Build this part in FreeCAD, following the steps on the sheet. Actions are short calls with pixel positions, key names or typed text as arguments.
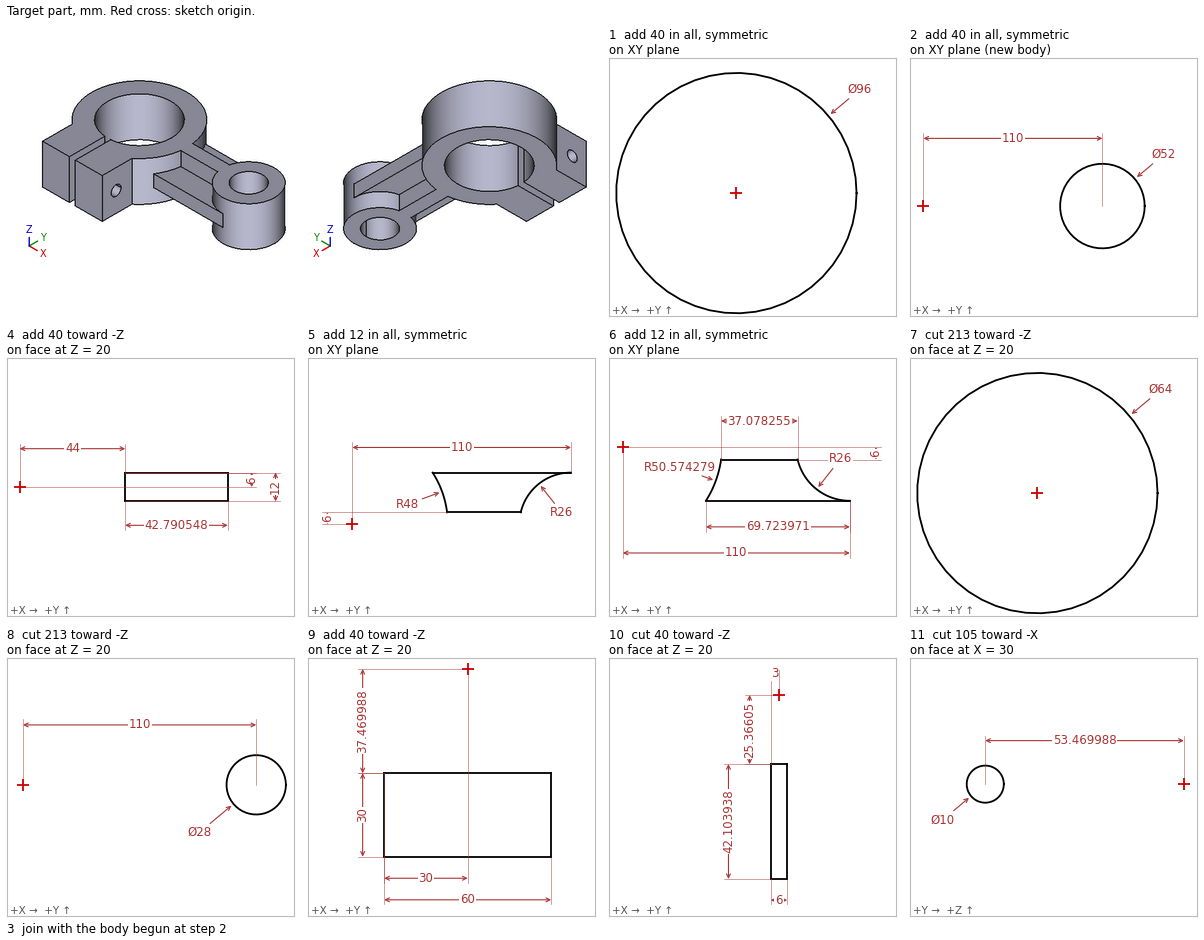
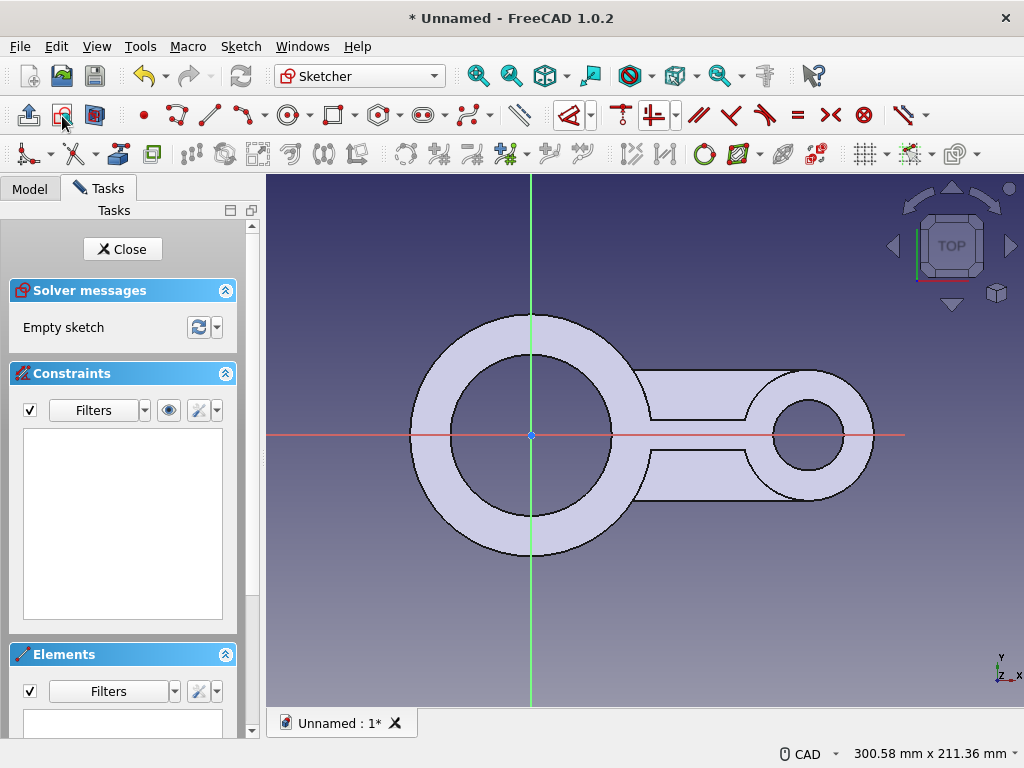
scroll(476, 618, up, 3)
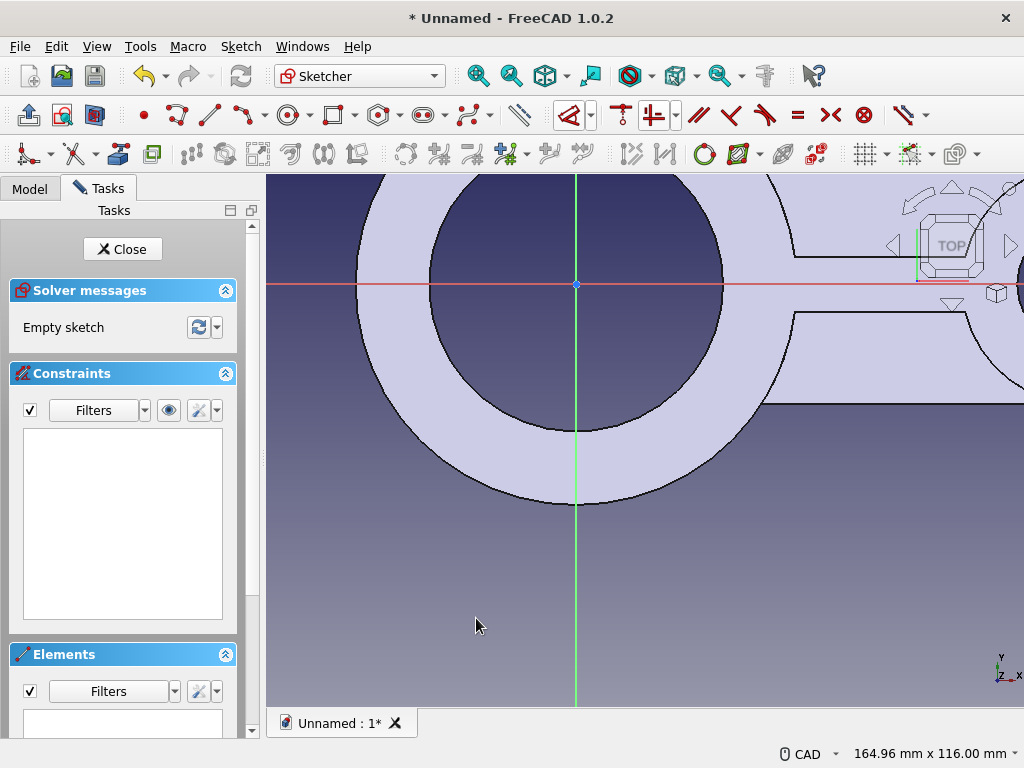
click(332, 116)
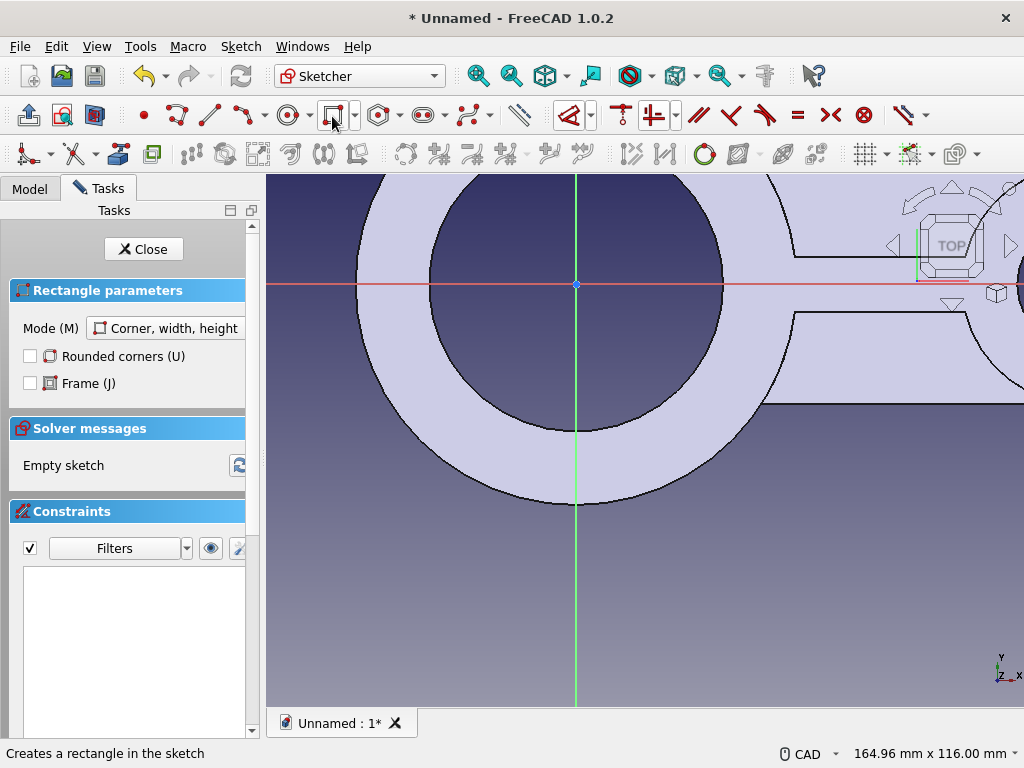
click(438, 457)
click(714, 594)
key(Escape)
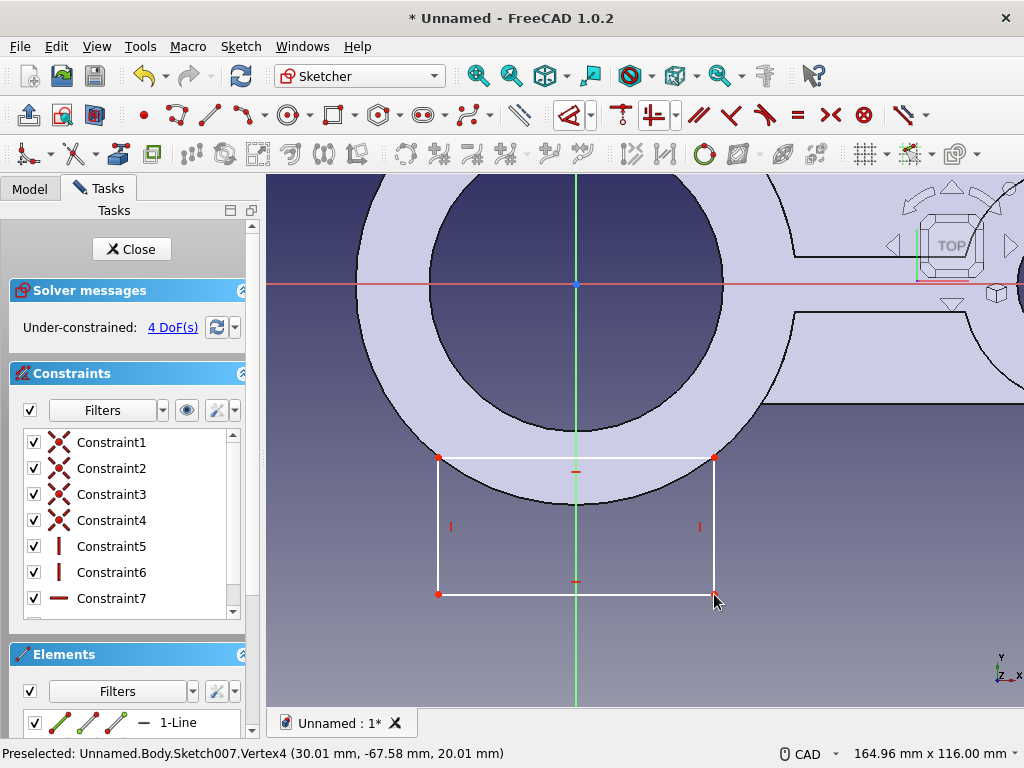
click(438, 499)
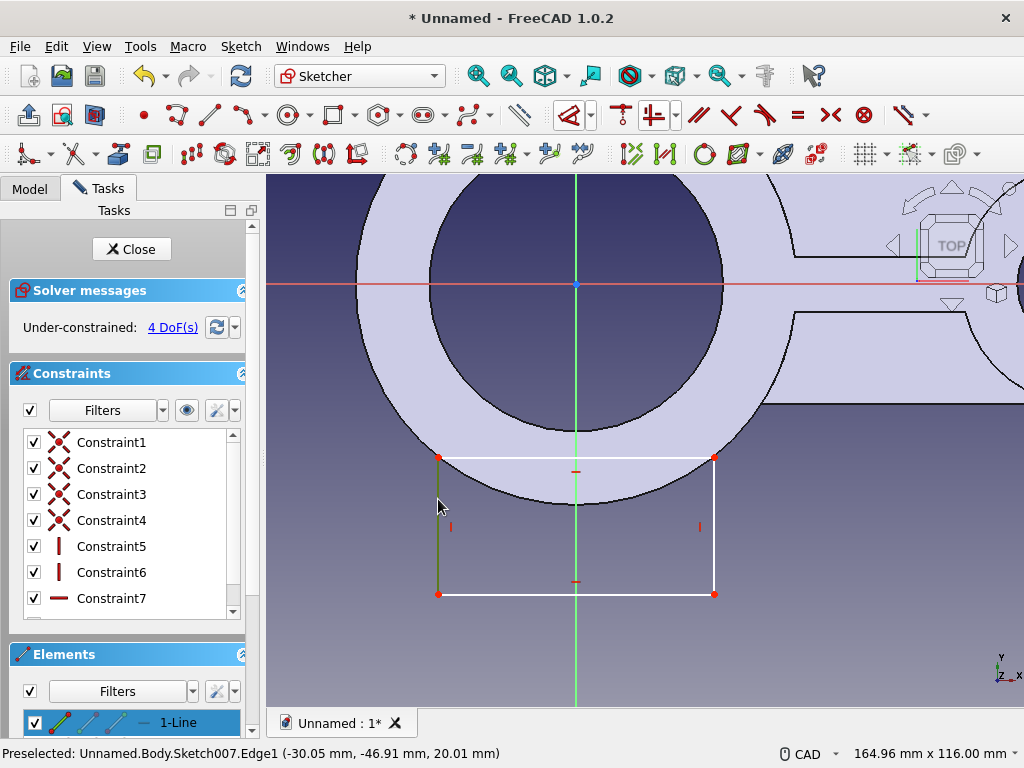
key(i)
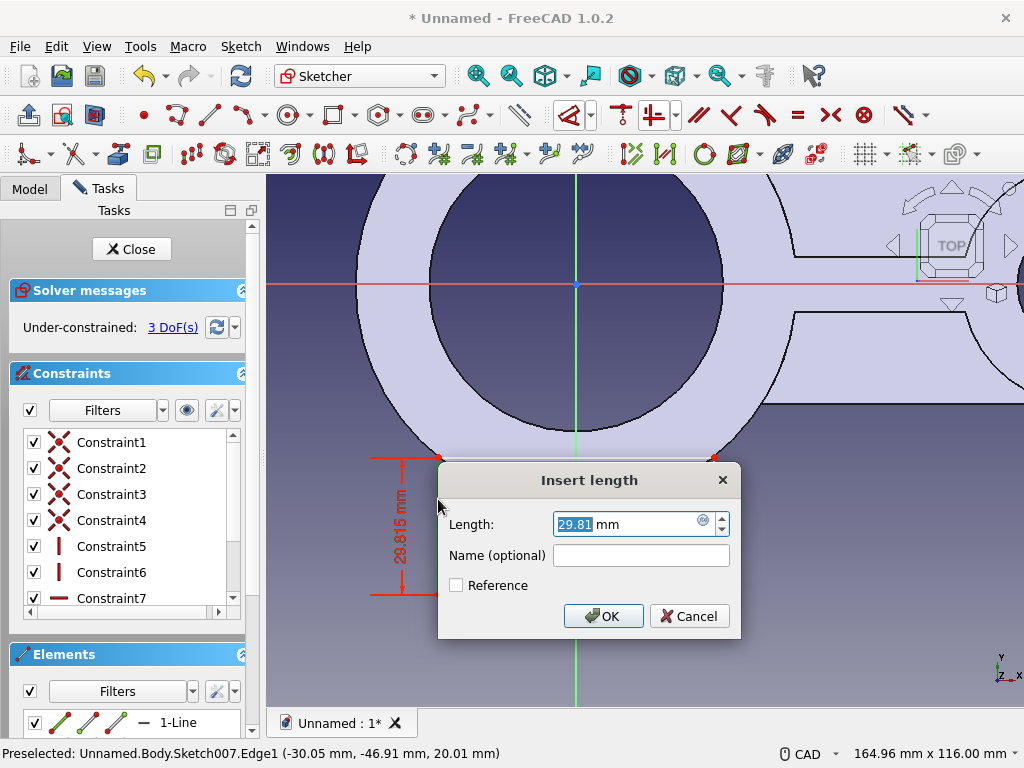
text(30)
key(Return)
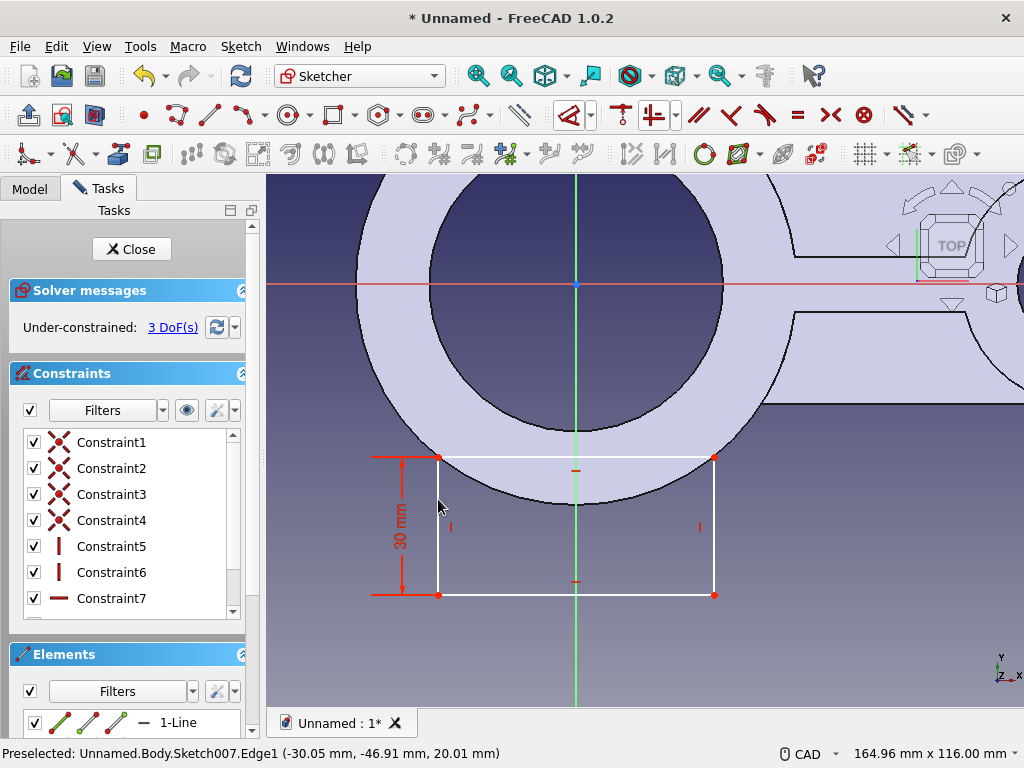
click(521, 595)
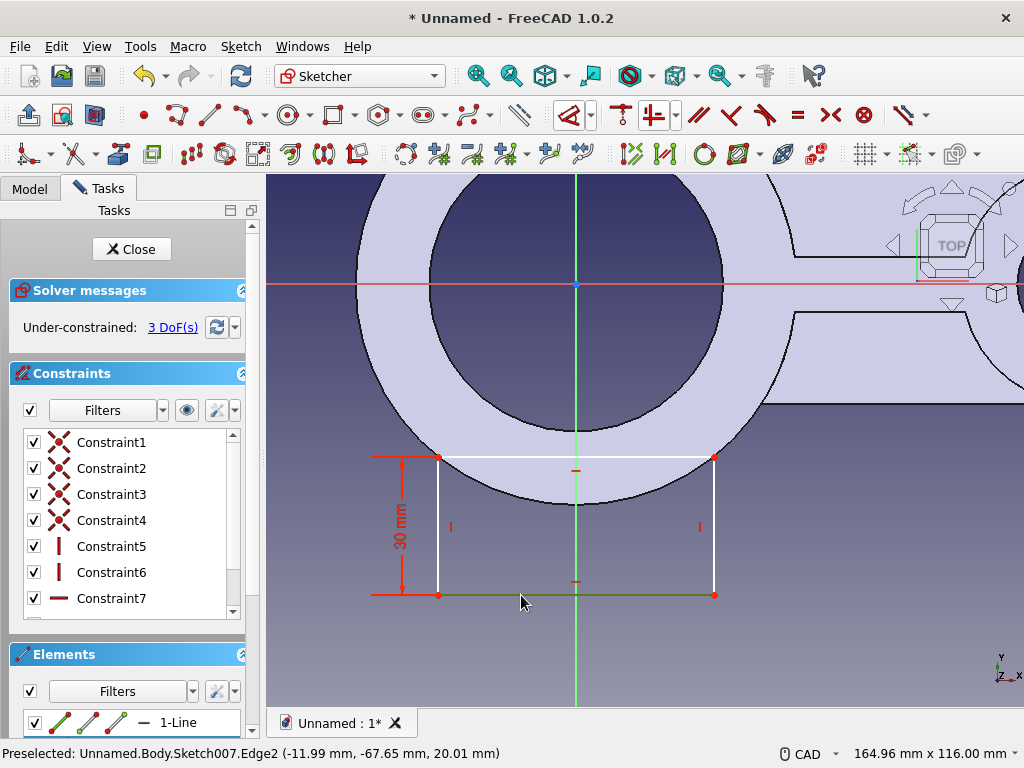
click(590, 116)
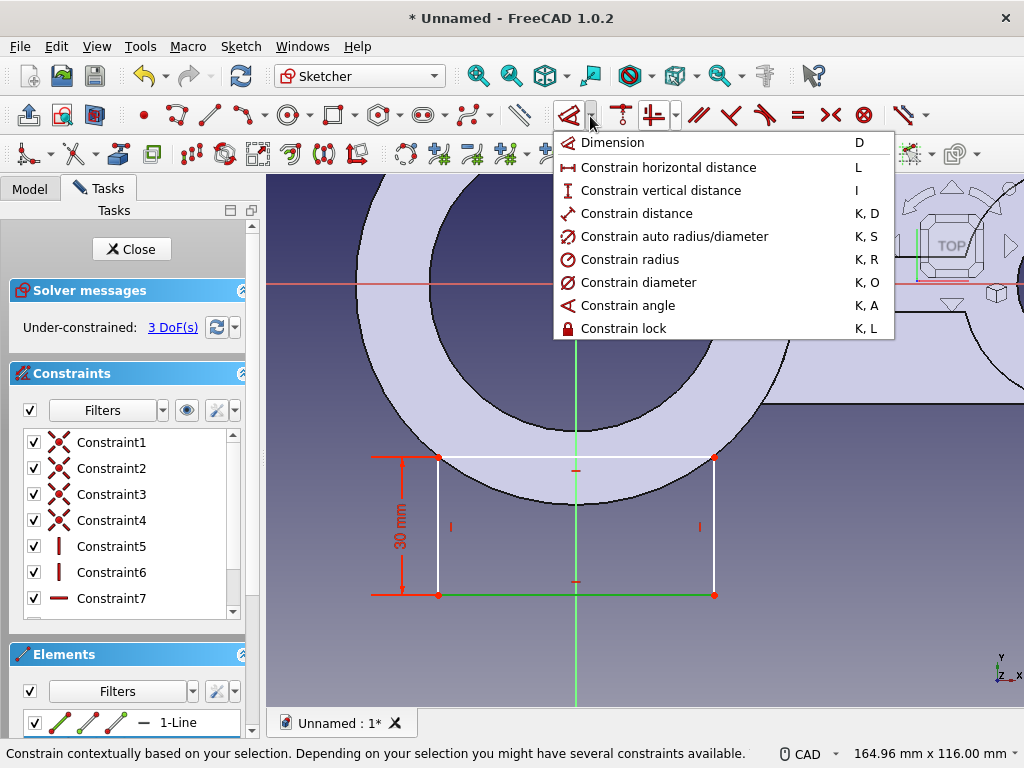
click(724, 168)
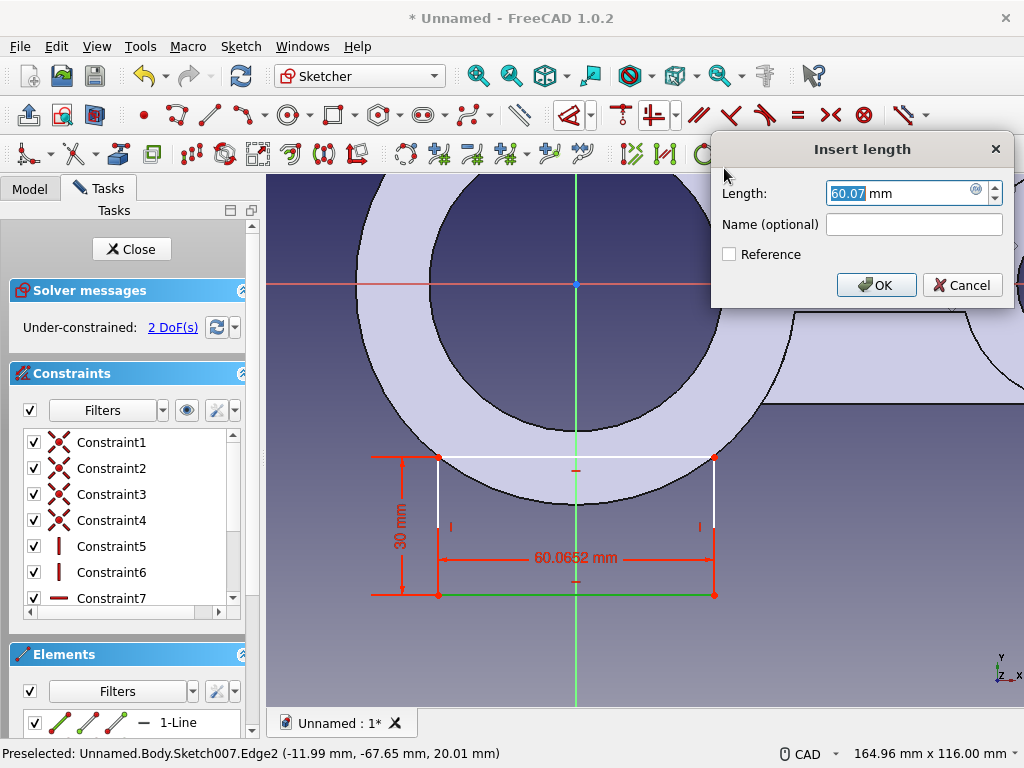
text(60)
key(Return)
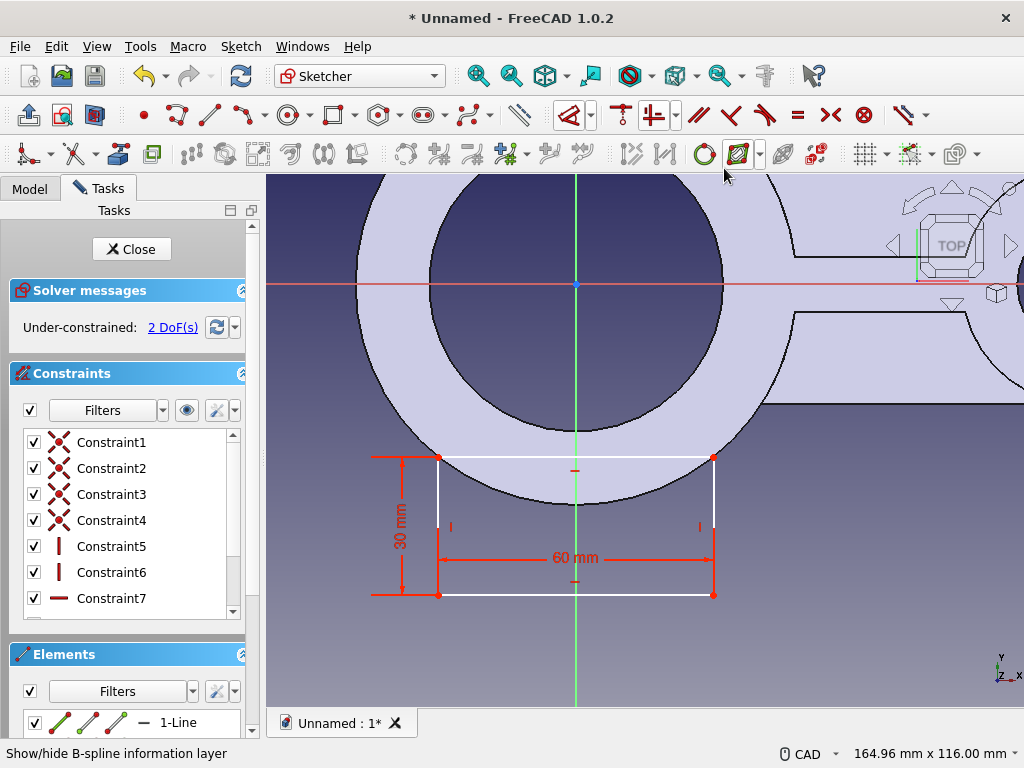
click(438, 457)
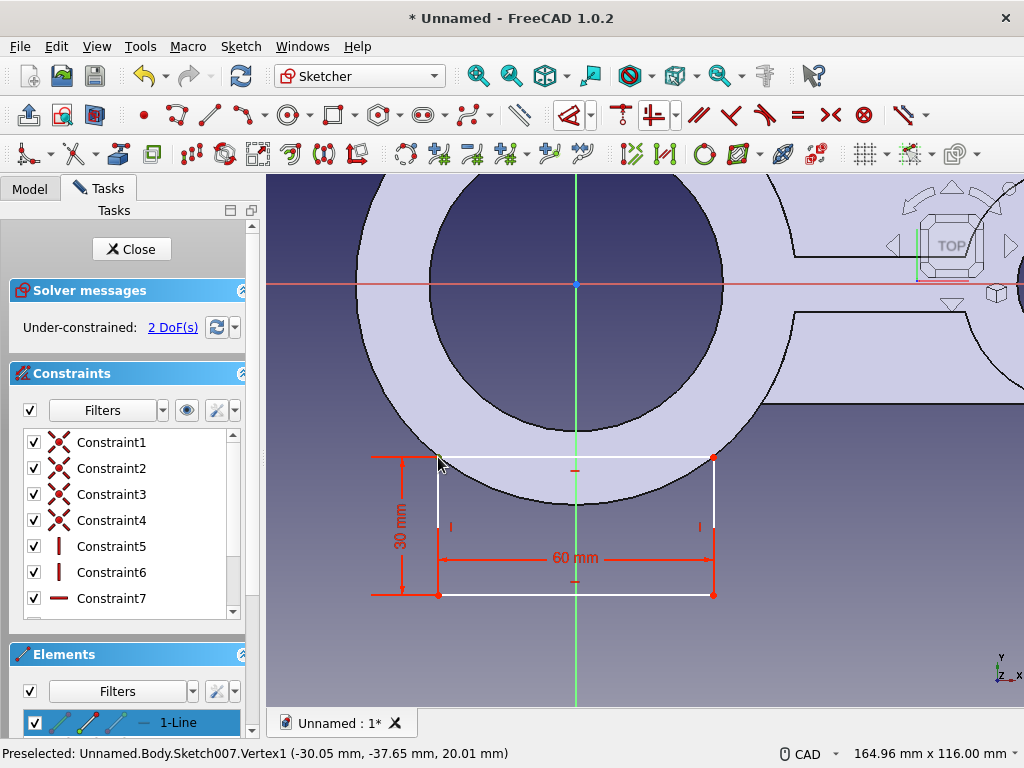
key(l)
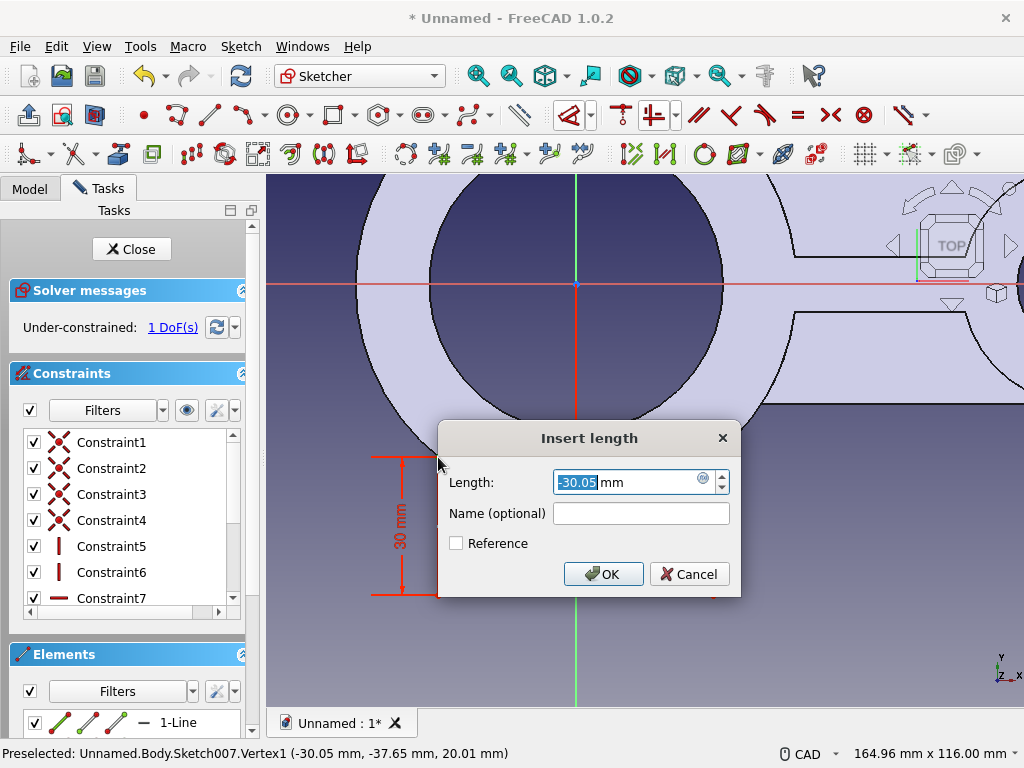
text(-30)
key(Return)